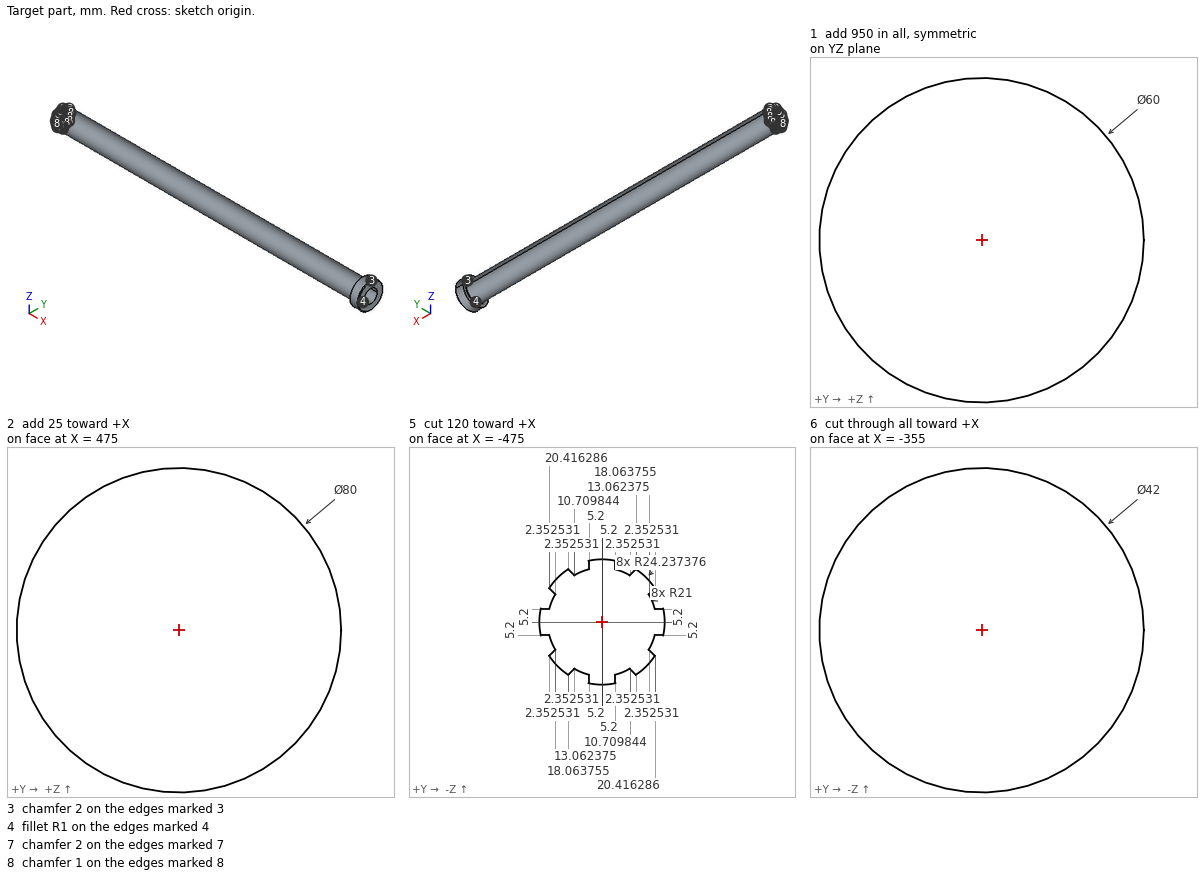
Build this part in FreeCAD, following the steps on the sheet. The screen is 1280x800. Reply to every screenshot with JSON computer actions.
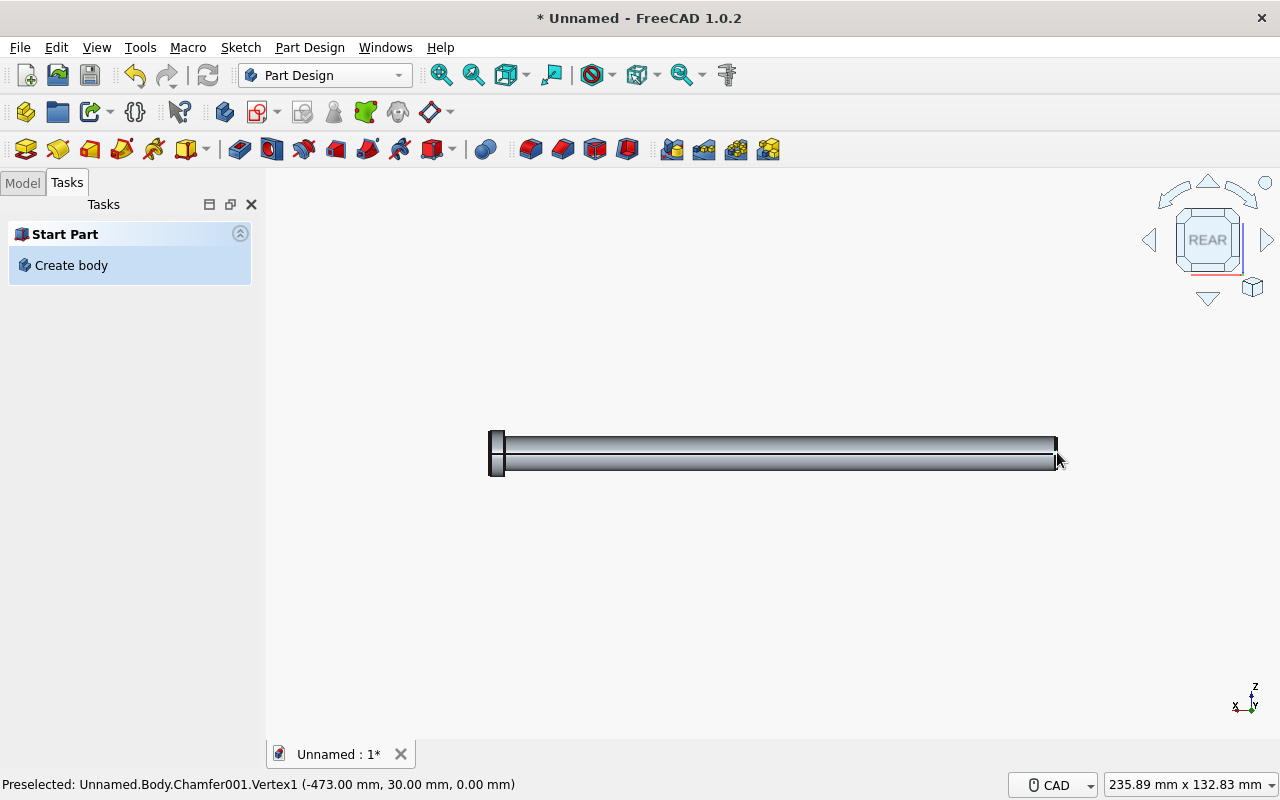
{"action": "key", "text": "6"}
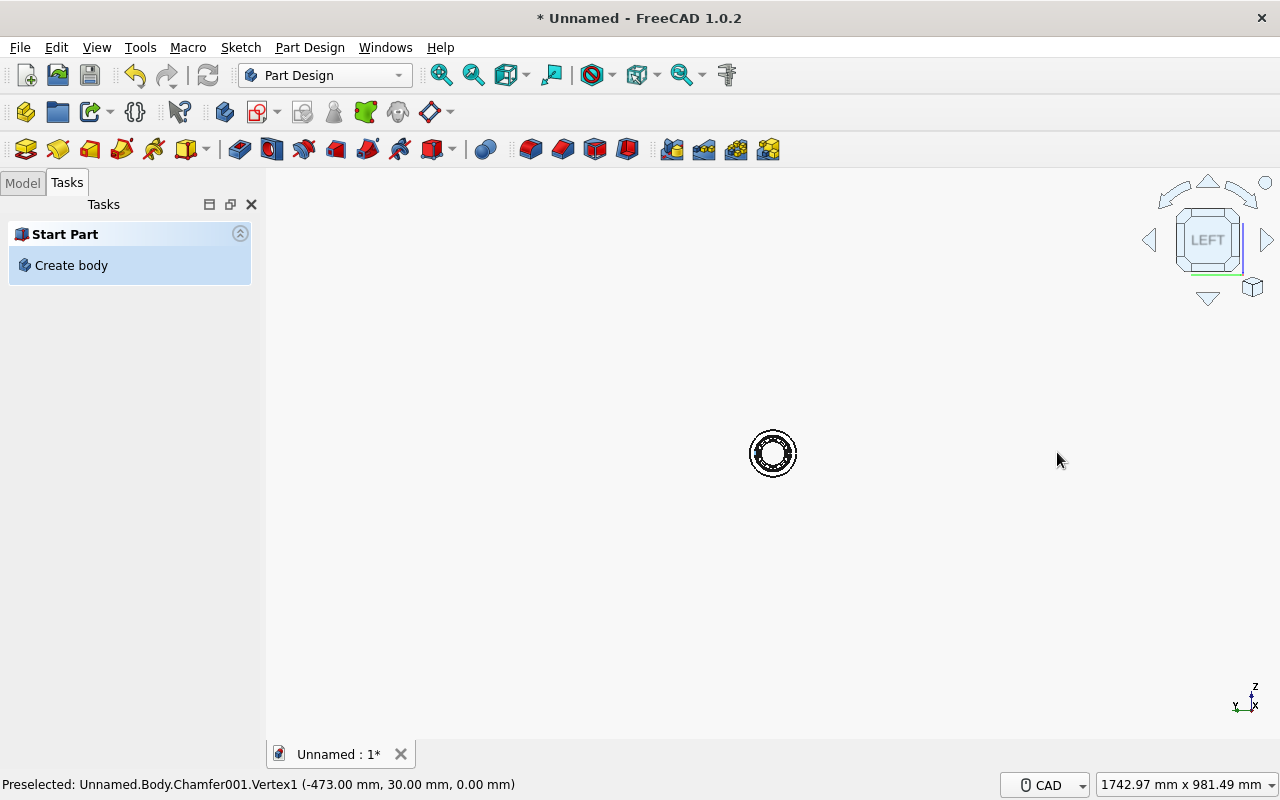
{"action": "left_click", "coordinate": [442, 76]}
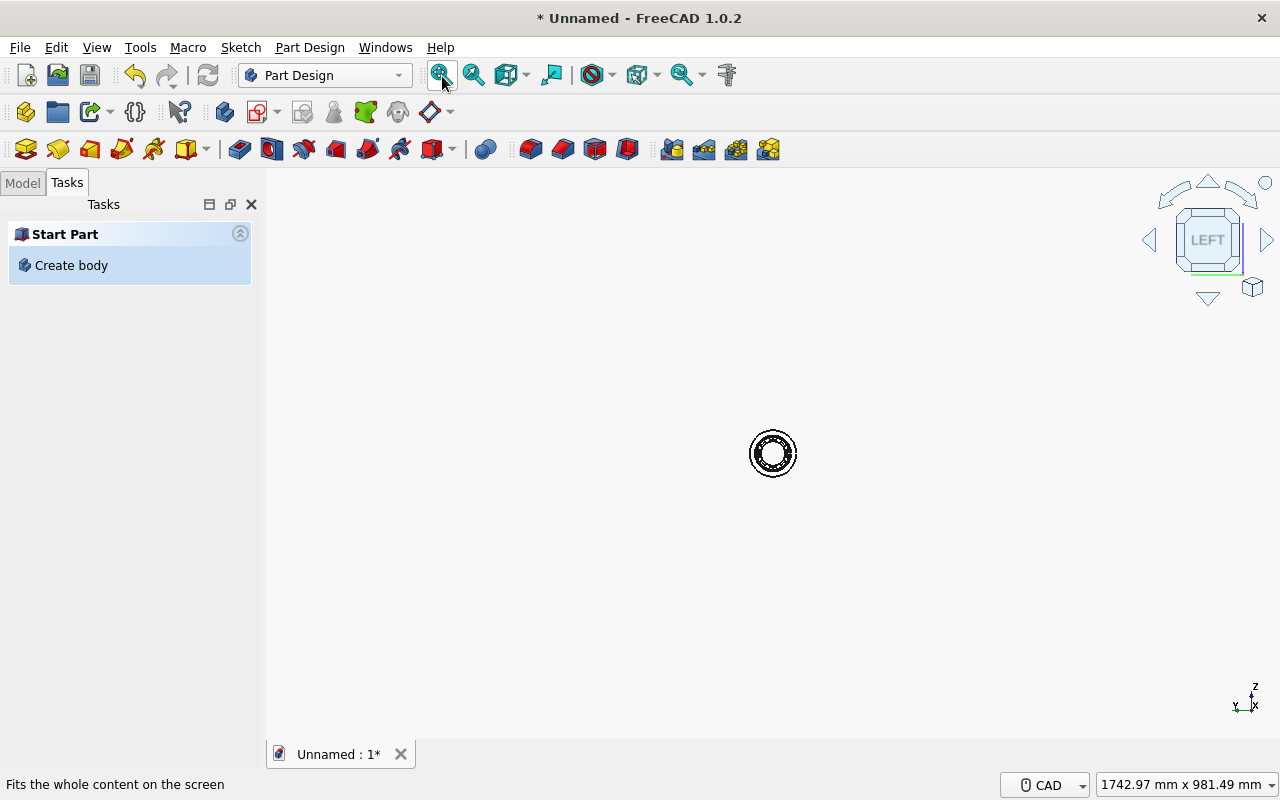
{"action": "scroll", "coordinate": [787, 452], "scroll_direction": "up", "scroll_amount": 10}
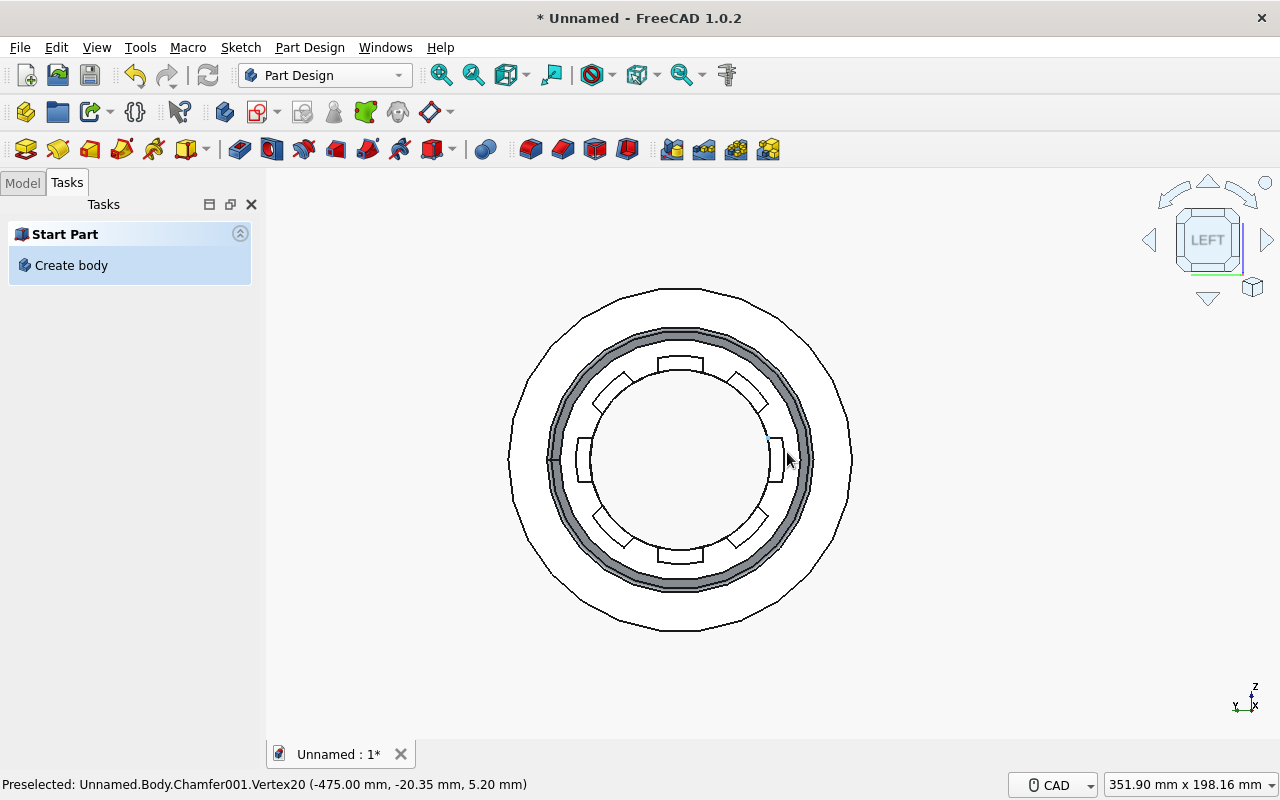
{"action": "left_click", "coordinate": [784, 459]}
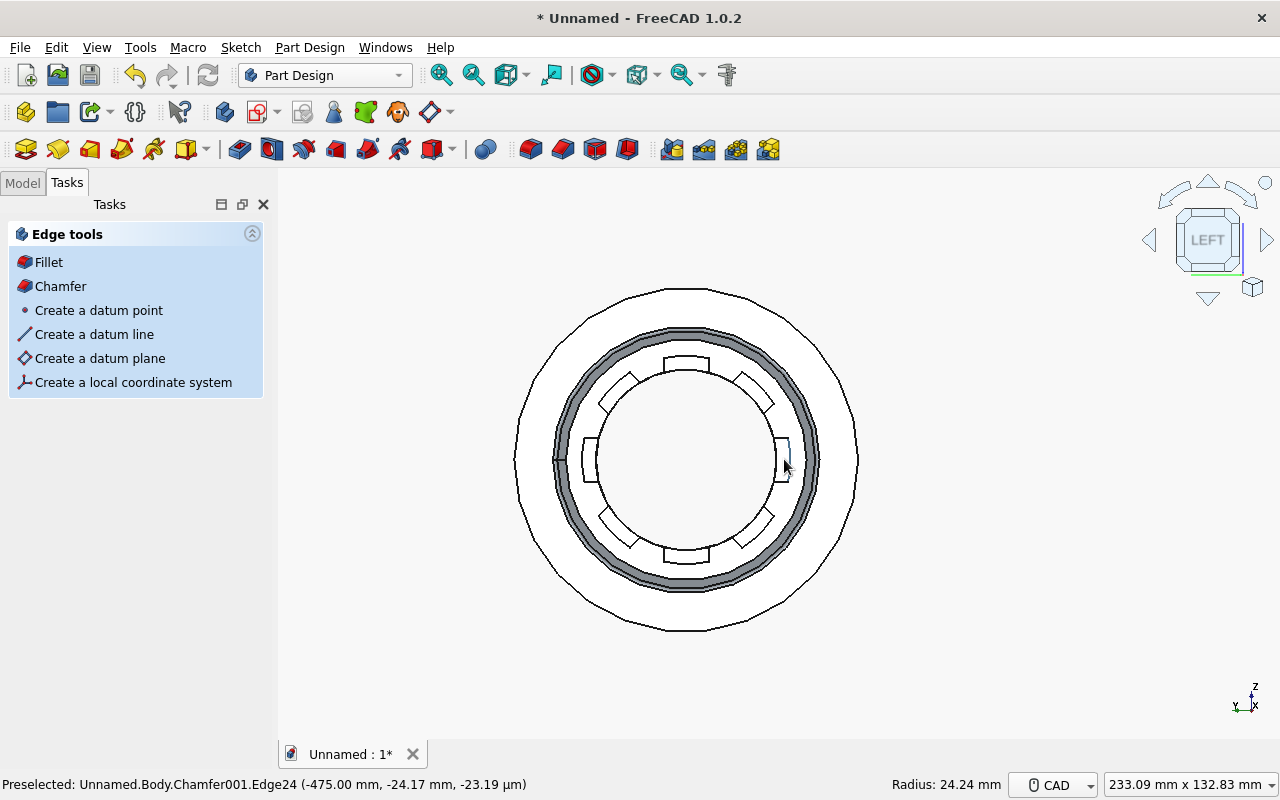
{"action": "left_click", "coordinate": [770, 424], "text": "ctrl"}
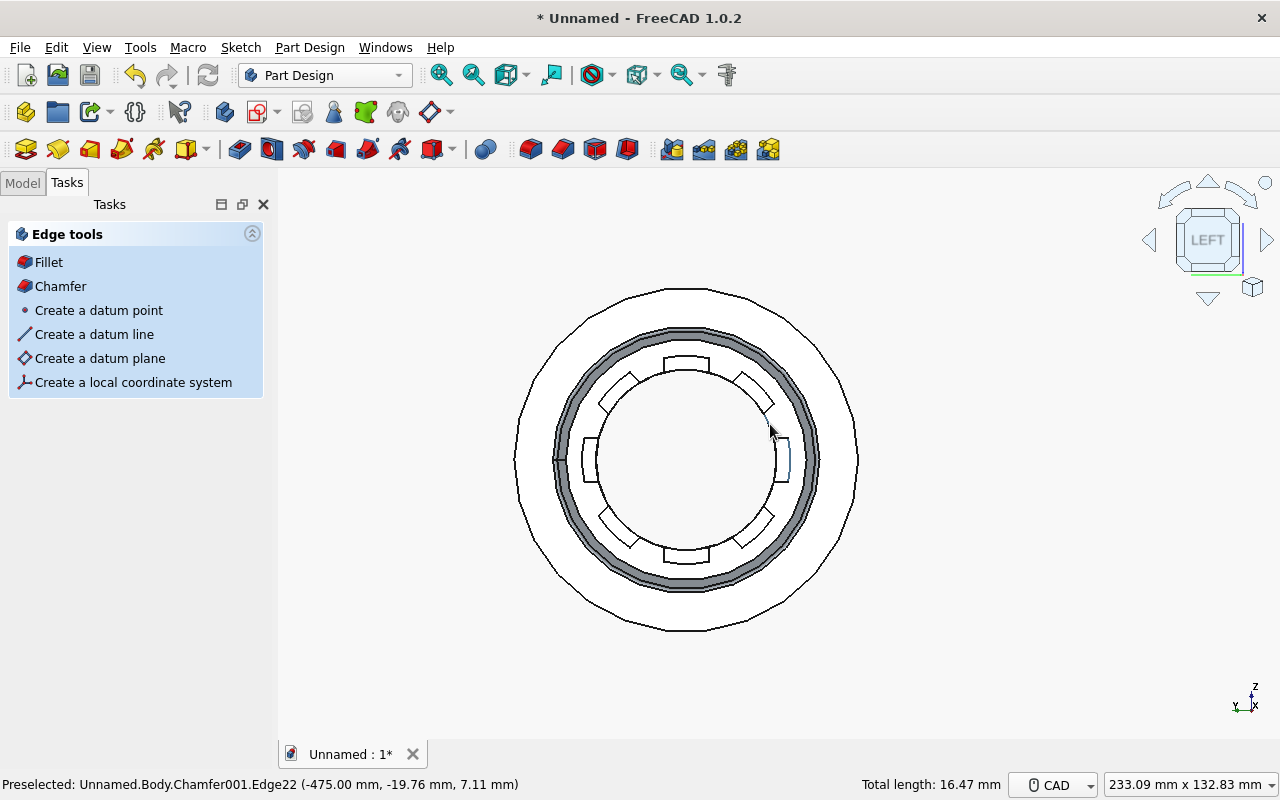
{"action": "left_click", "coordinate": [760, 385], "text": "ctrl"}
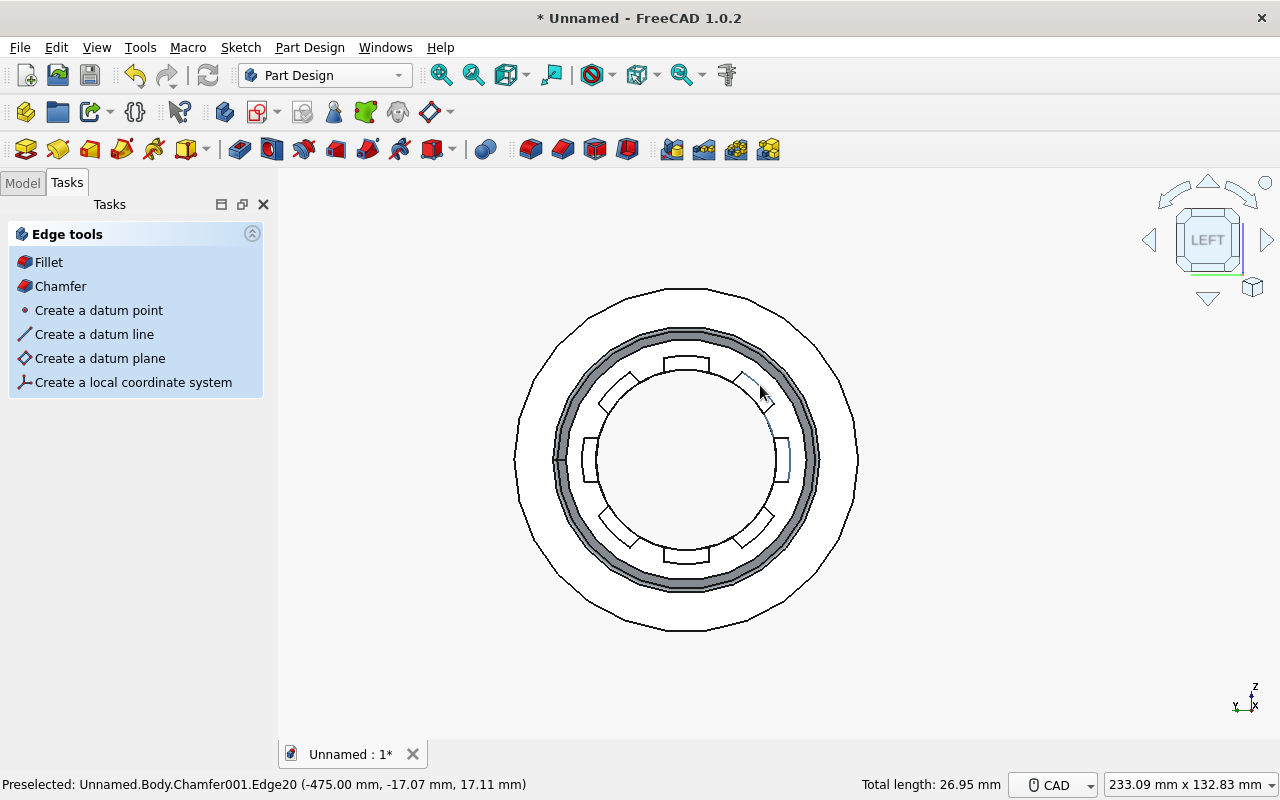
{"action": "left_click", "coordinate": [721, 375], "text": "ctrl"}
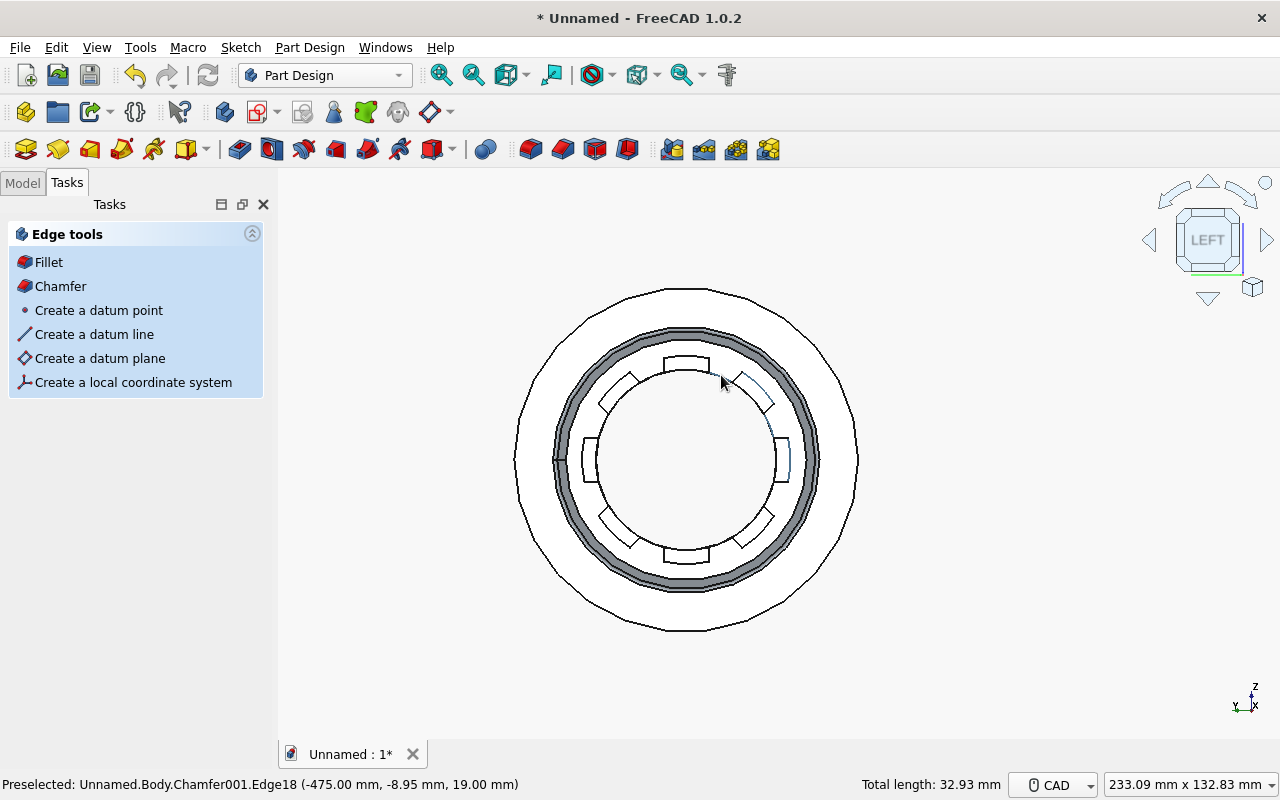
{"action": "left_click", "coordinate": [686, 355], "text": "ctrl"}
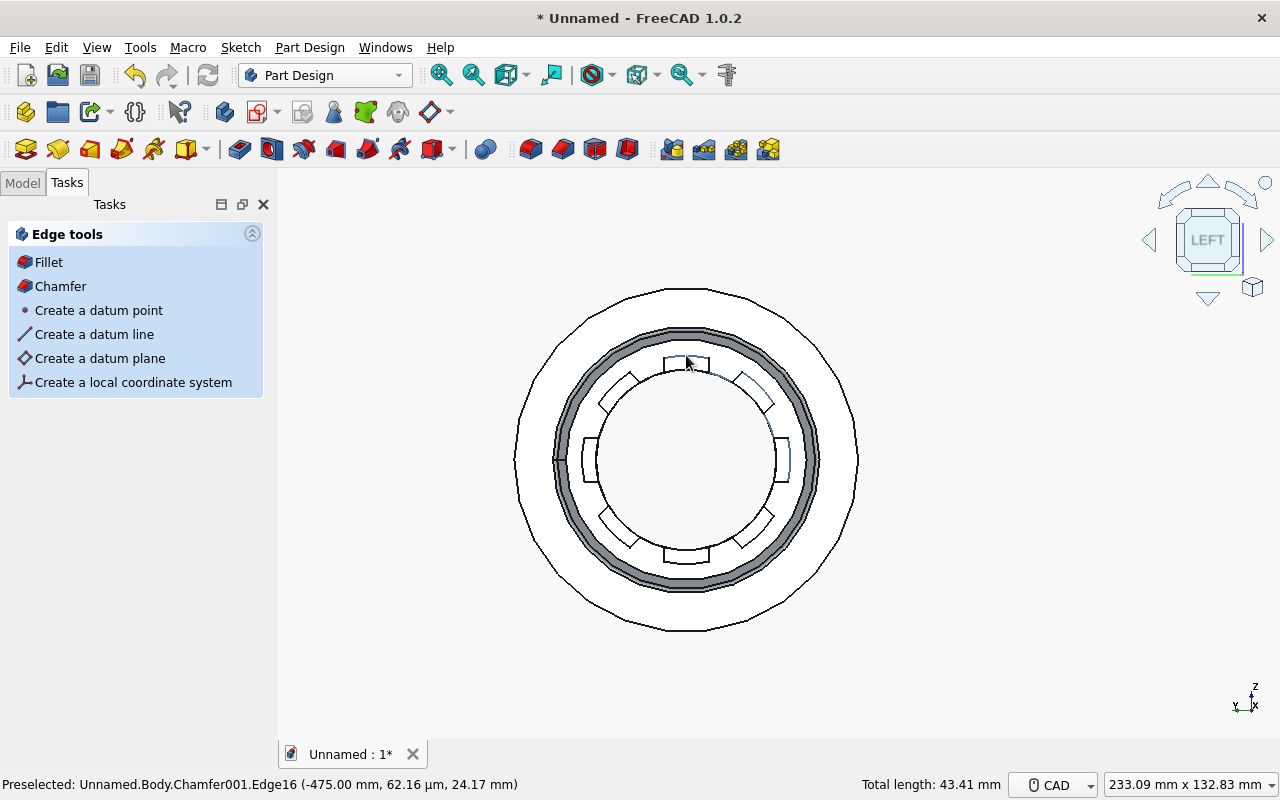
{"action": "left_click", "coordinate": [652, 375], "text": "ctrl"}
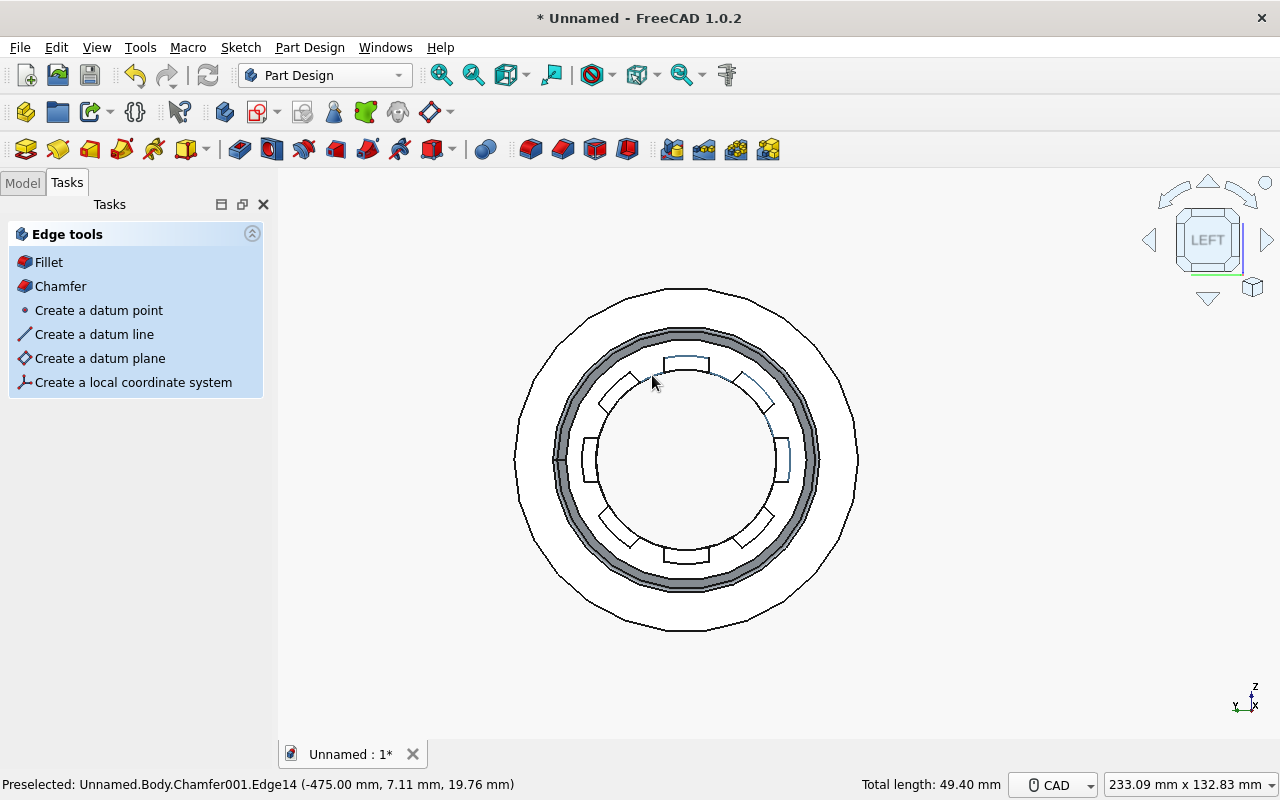
{"action": "left_click", "coordinate": [613, 385], "text": "ctrl"}